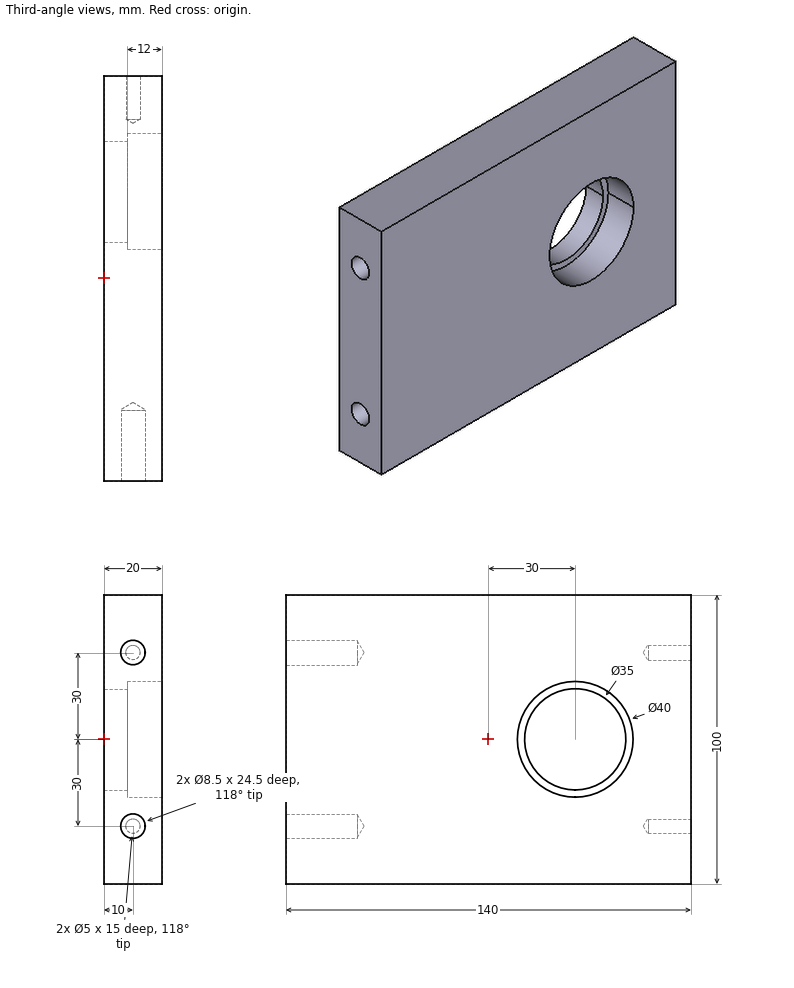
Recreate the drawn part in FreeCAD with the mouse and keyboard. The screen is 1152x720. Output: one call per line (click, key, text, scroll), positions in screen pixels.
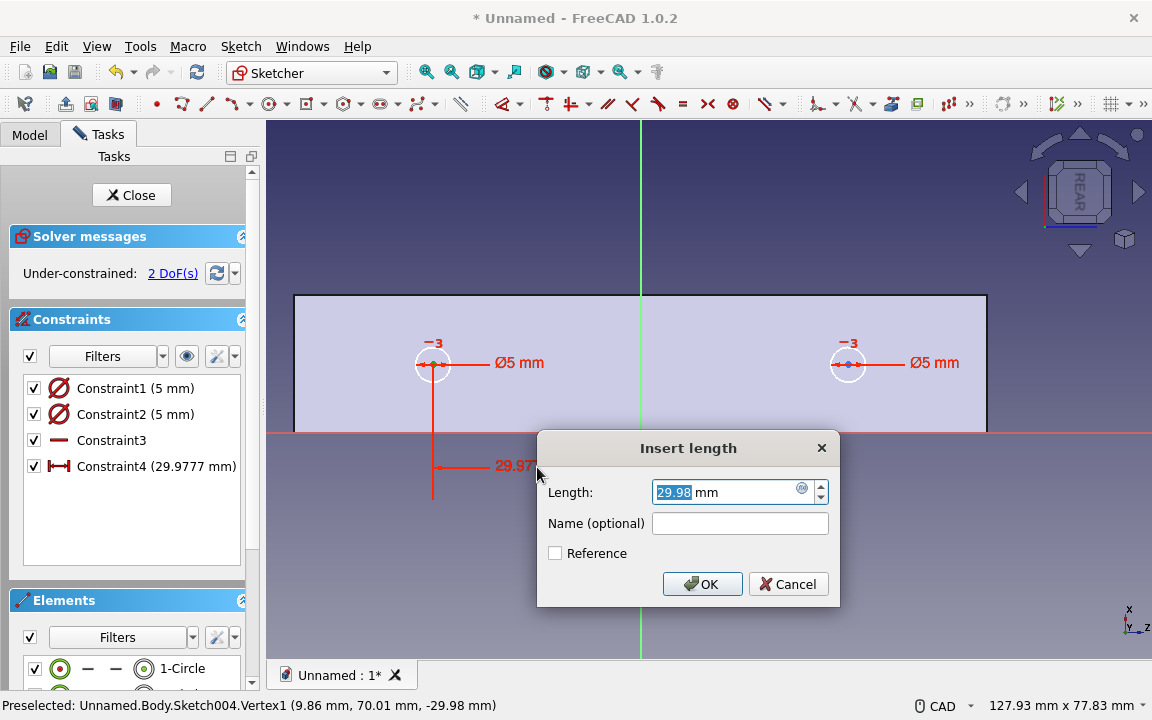
text(30)
key(Return)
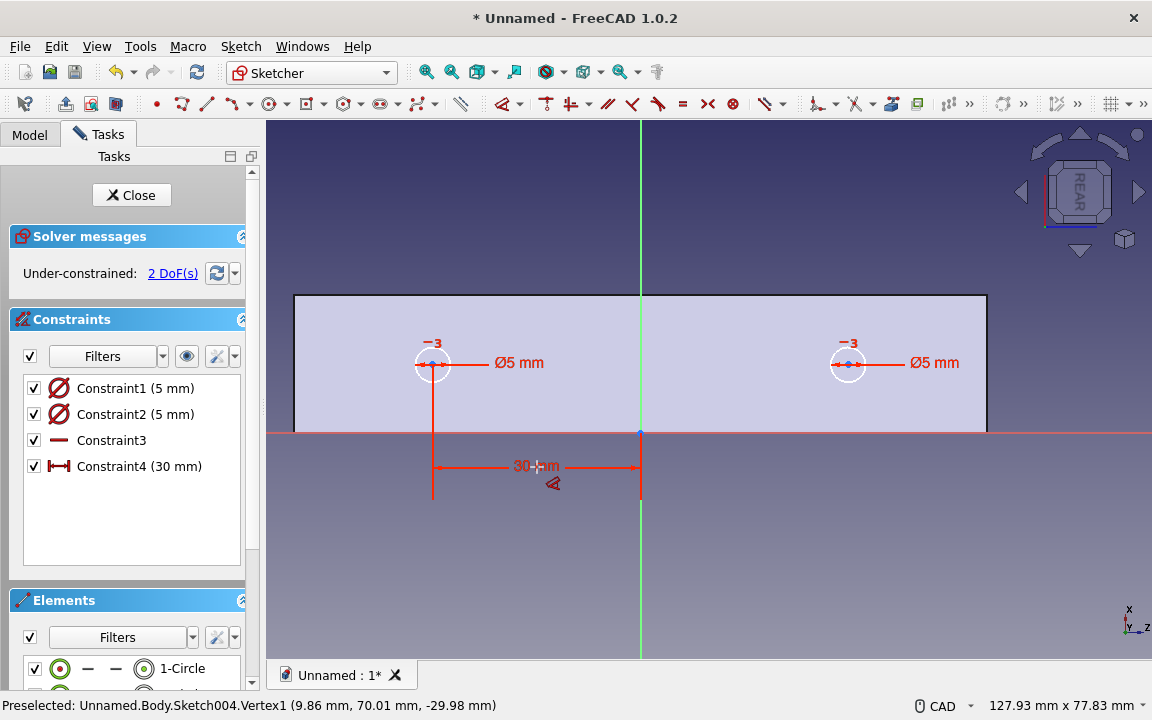
click(433, 365)
click(399, 399)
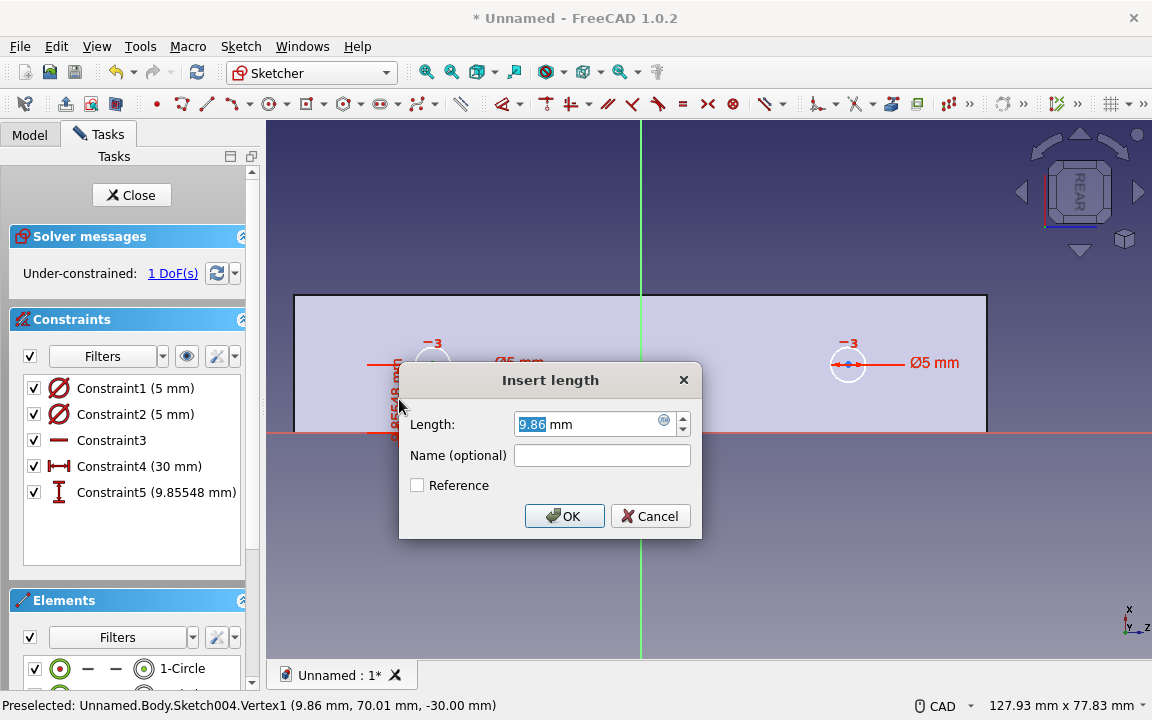
text(10)
key(Return)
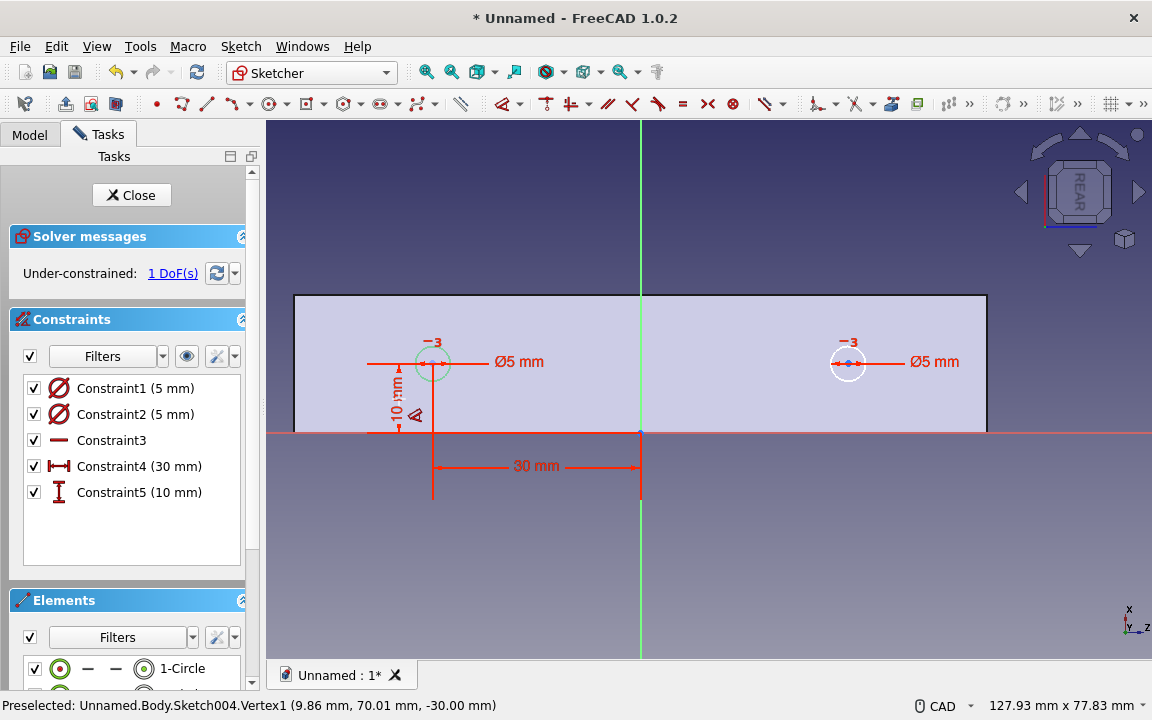
click(848, 364)
click(744, 467)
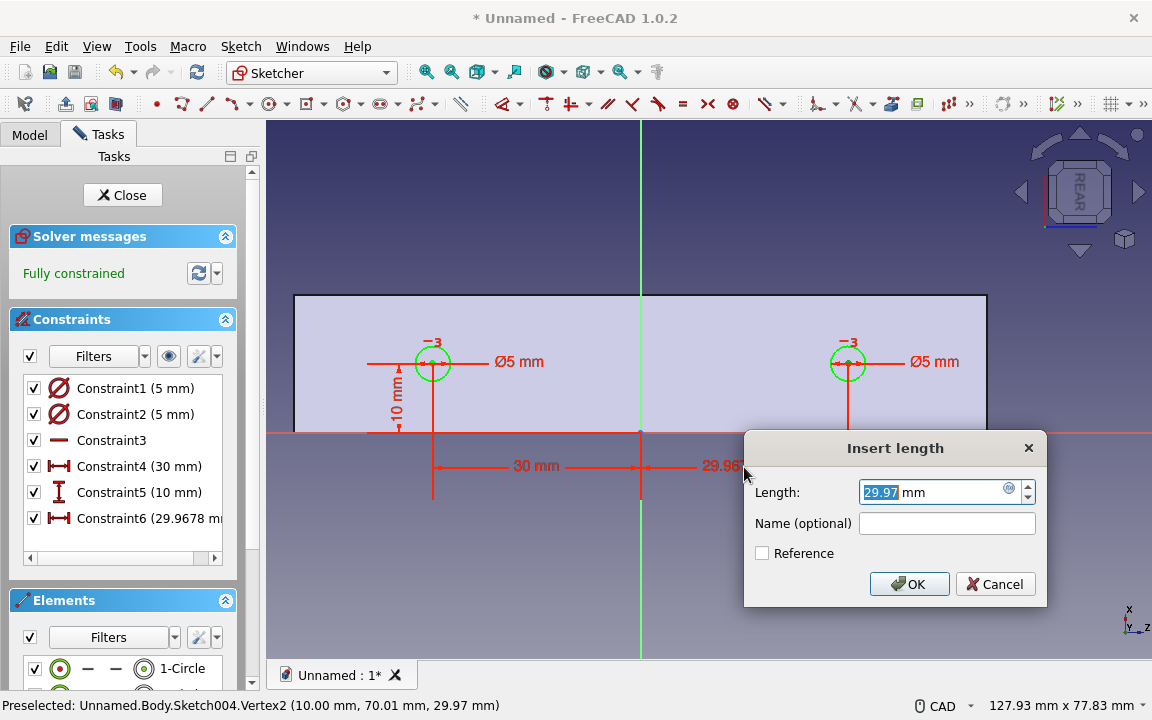
text(30)
key(Return)
key(Escape)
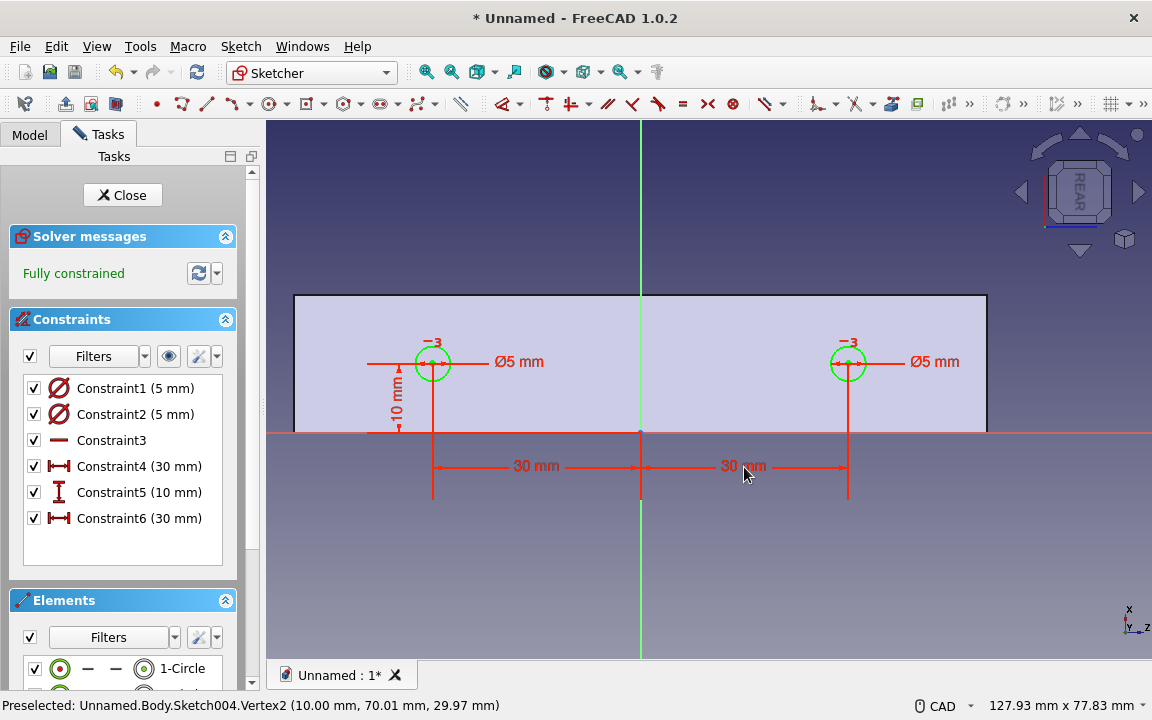
click(123, 195)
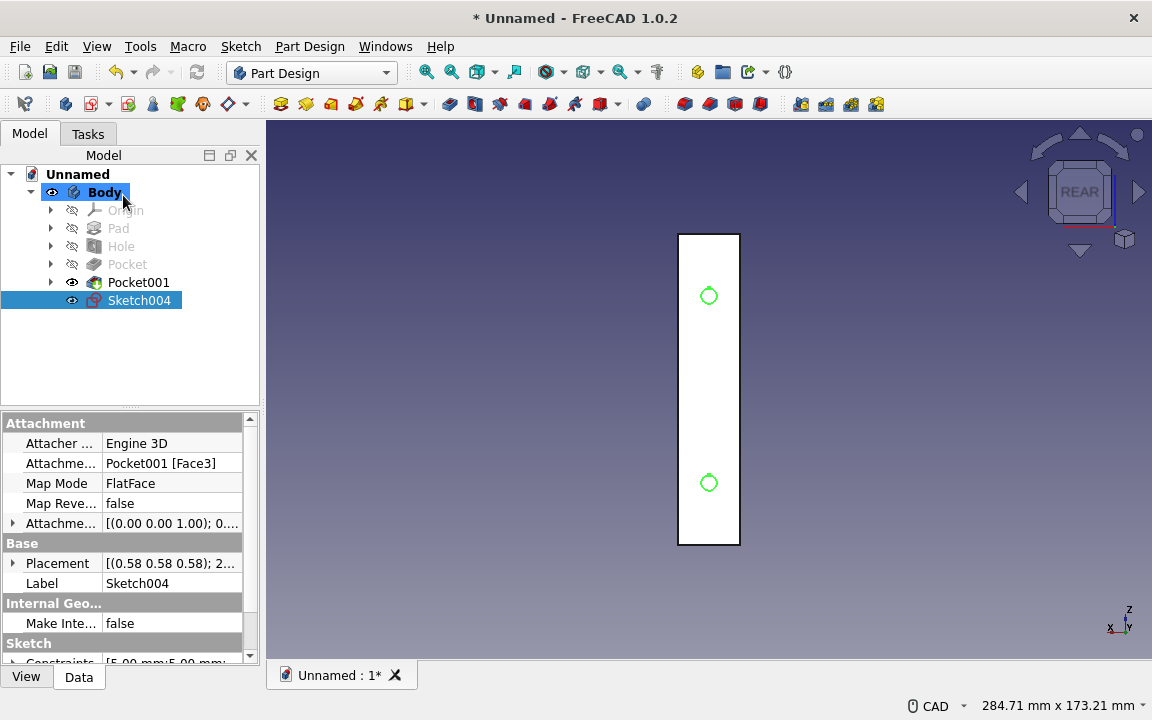
click(475, 104)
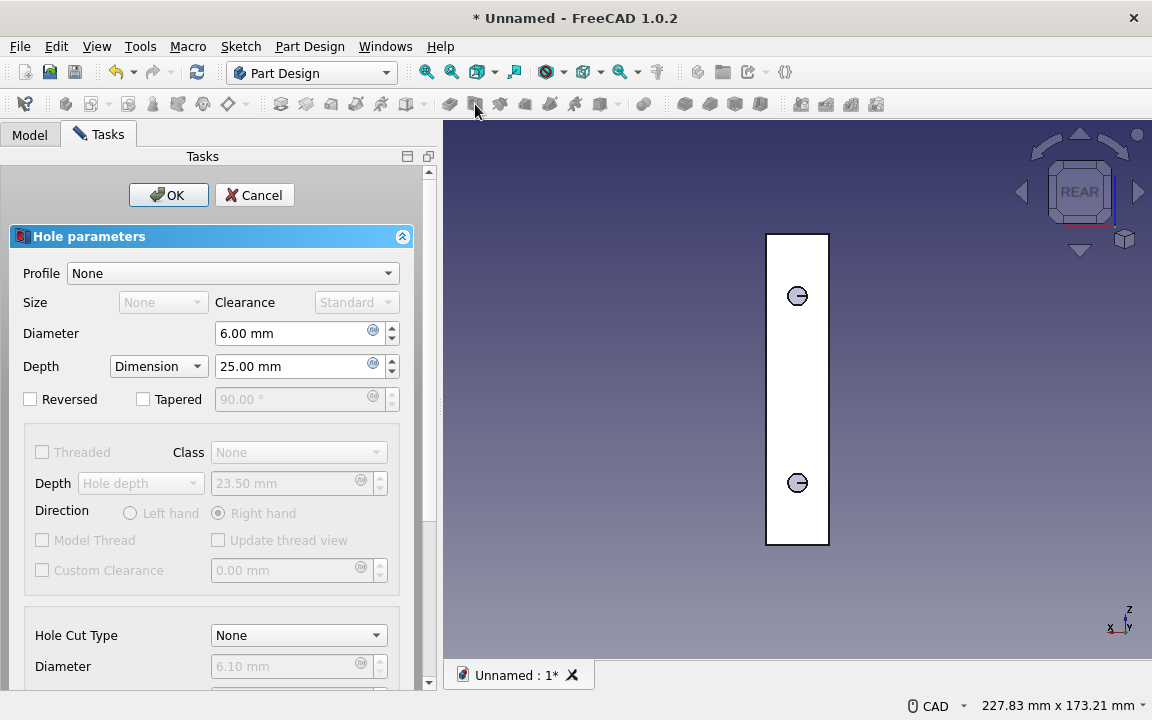
triple_click(300, 334)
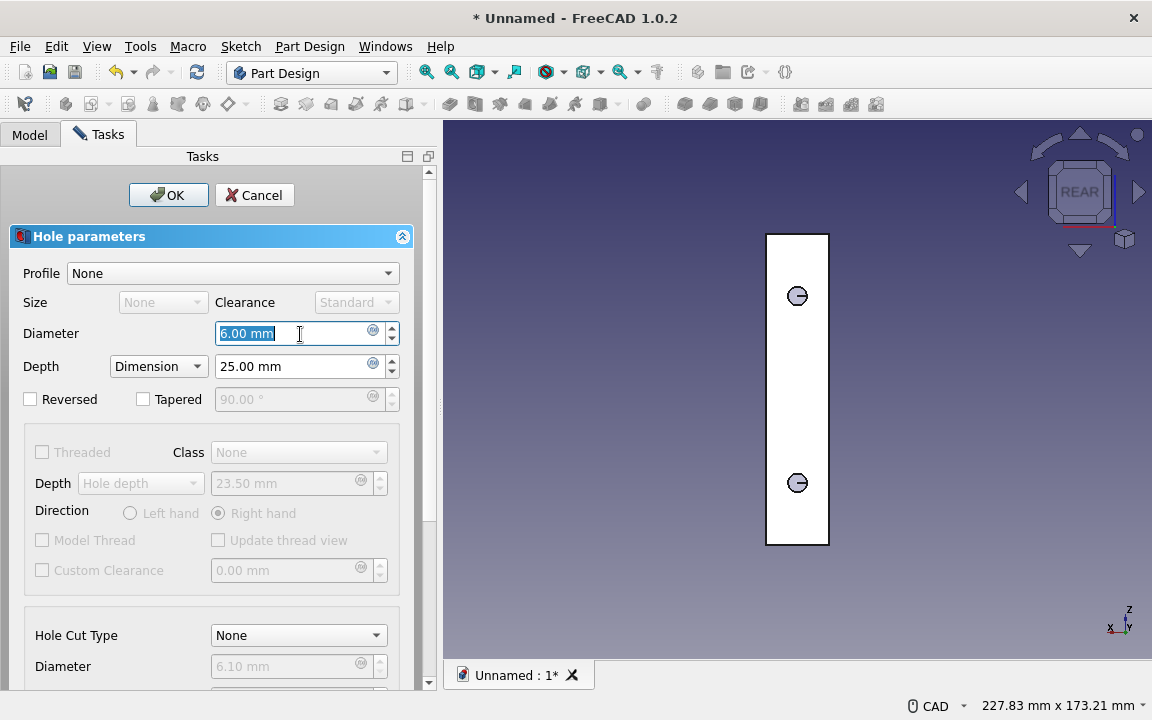
text(5)
key(Tab)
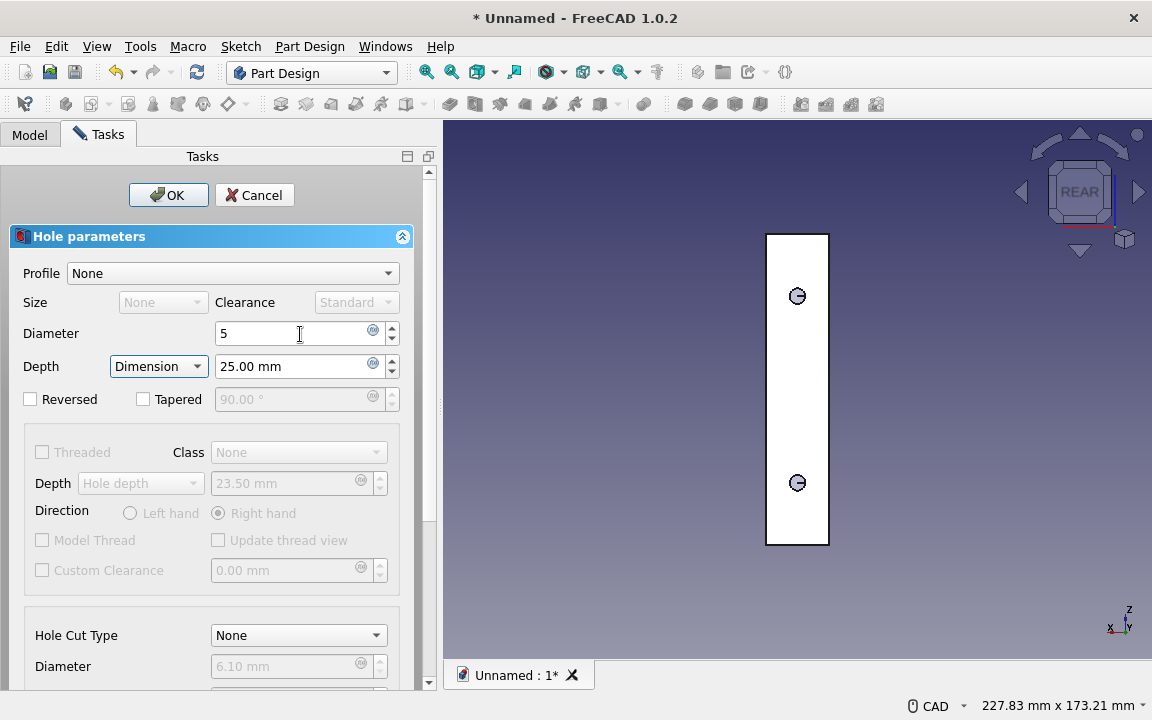
triple_click(300, 366)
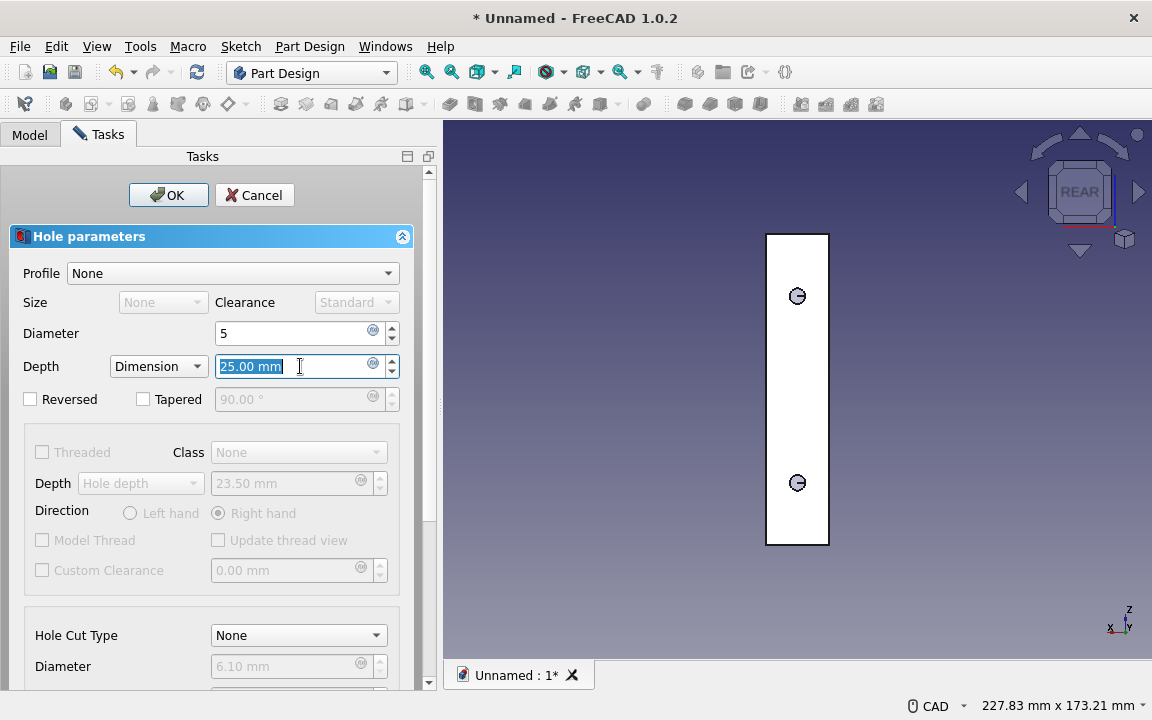
text(15)
key(Tab)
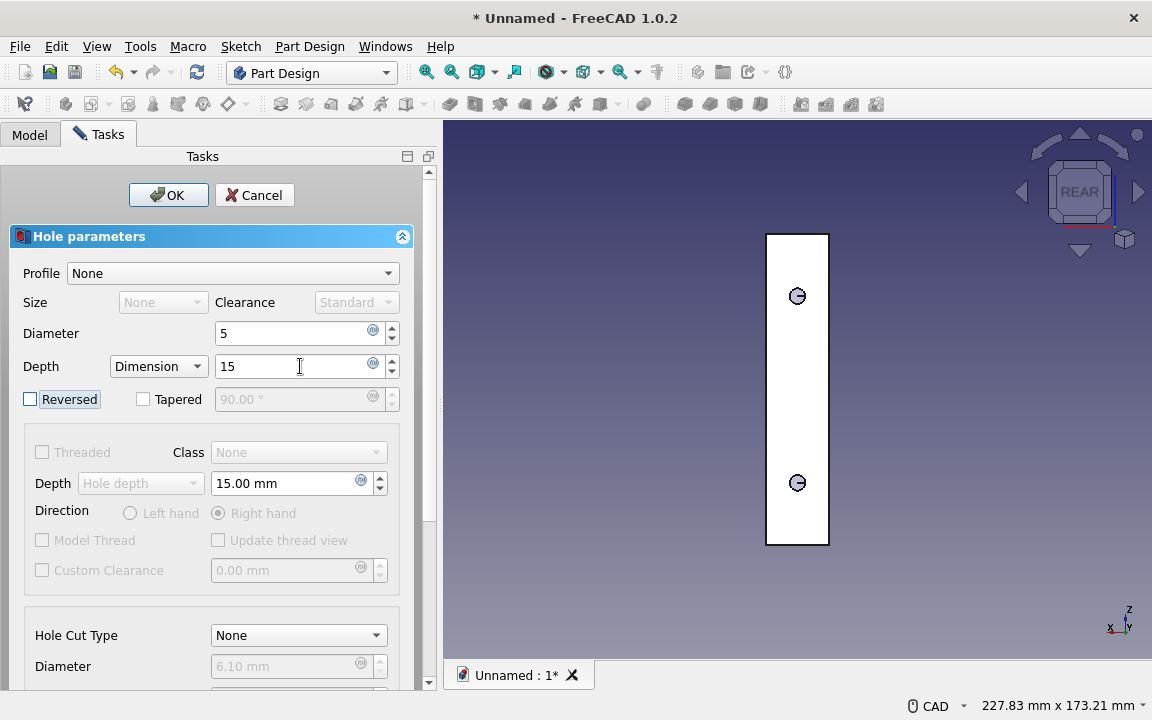
click(169, 195)